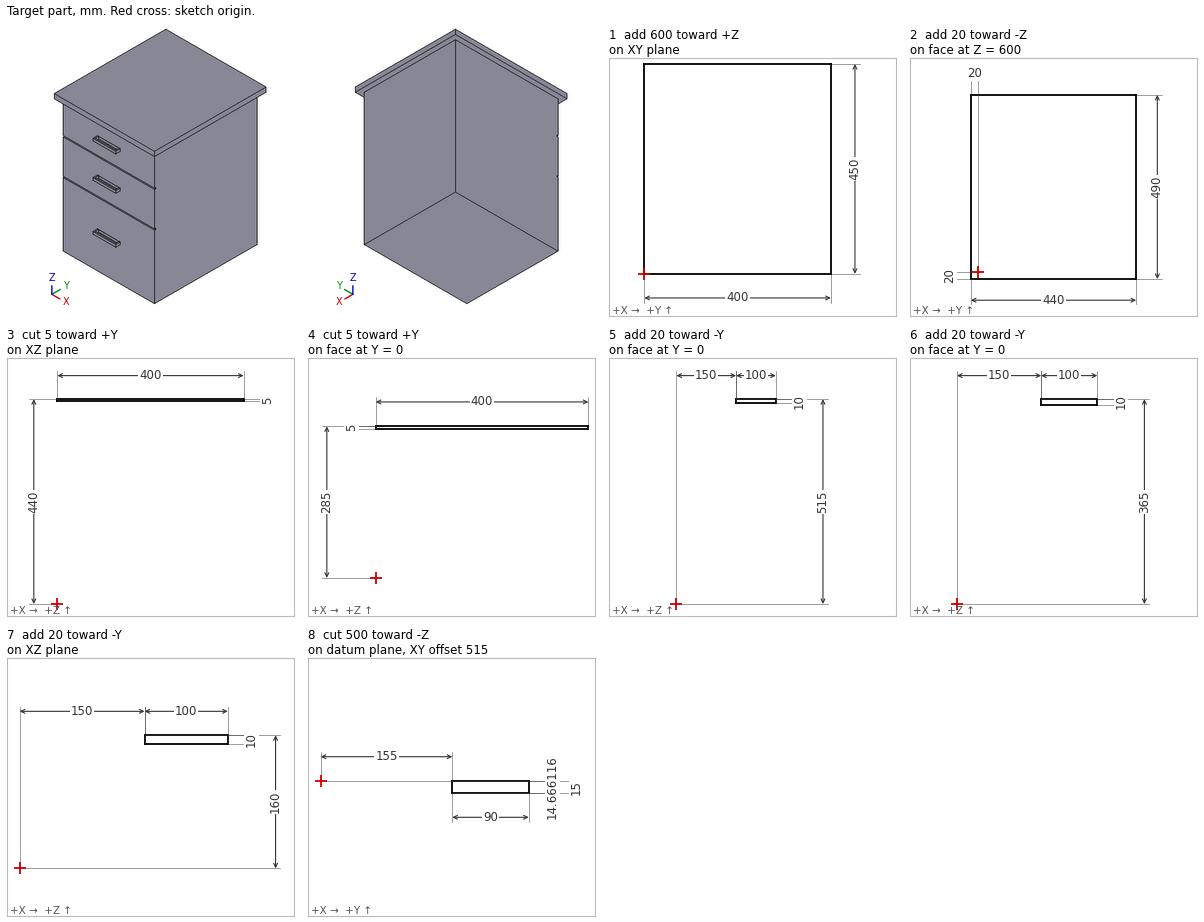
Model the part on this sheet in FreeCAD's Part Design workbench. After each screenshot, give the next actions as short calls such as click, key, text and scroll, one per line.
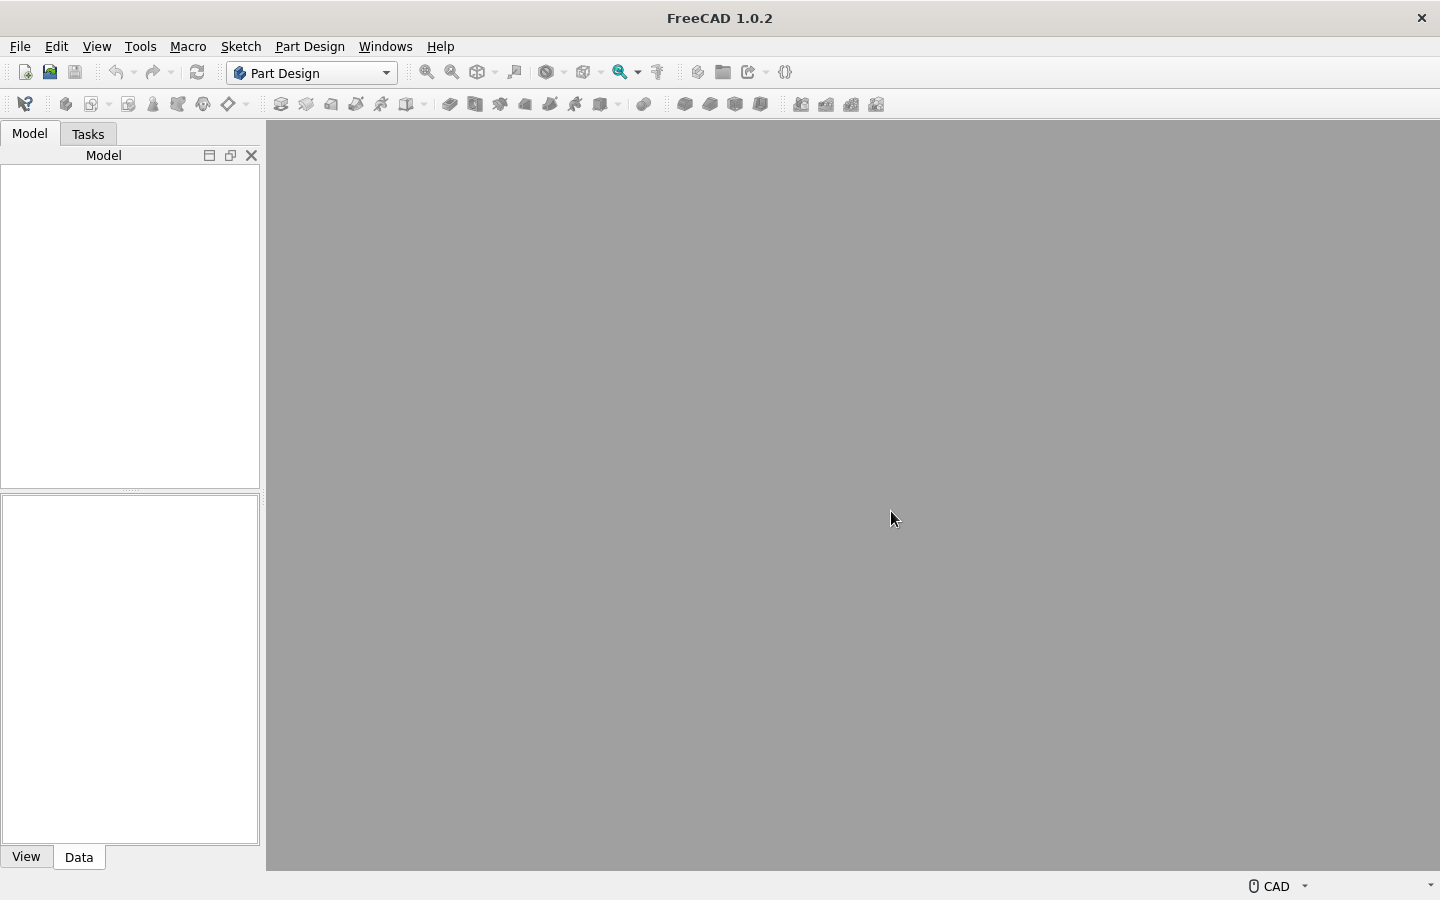
click(25, 72)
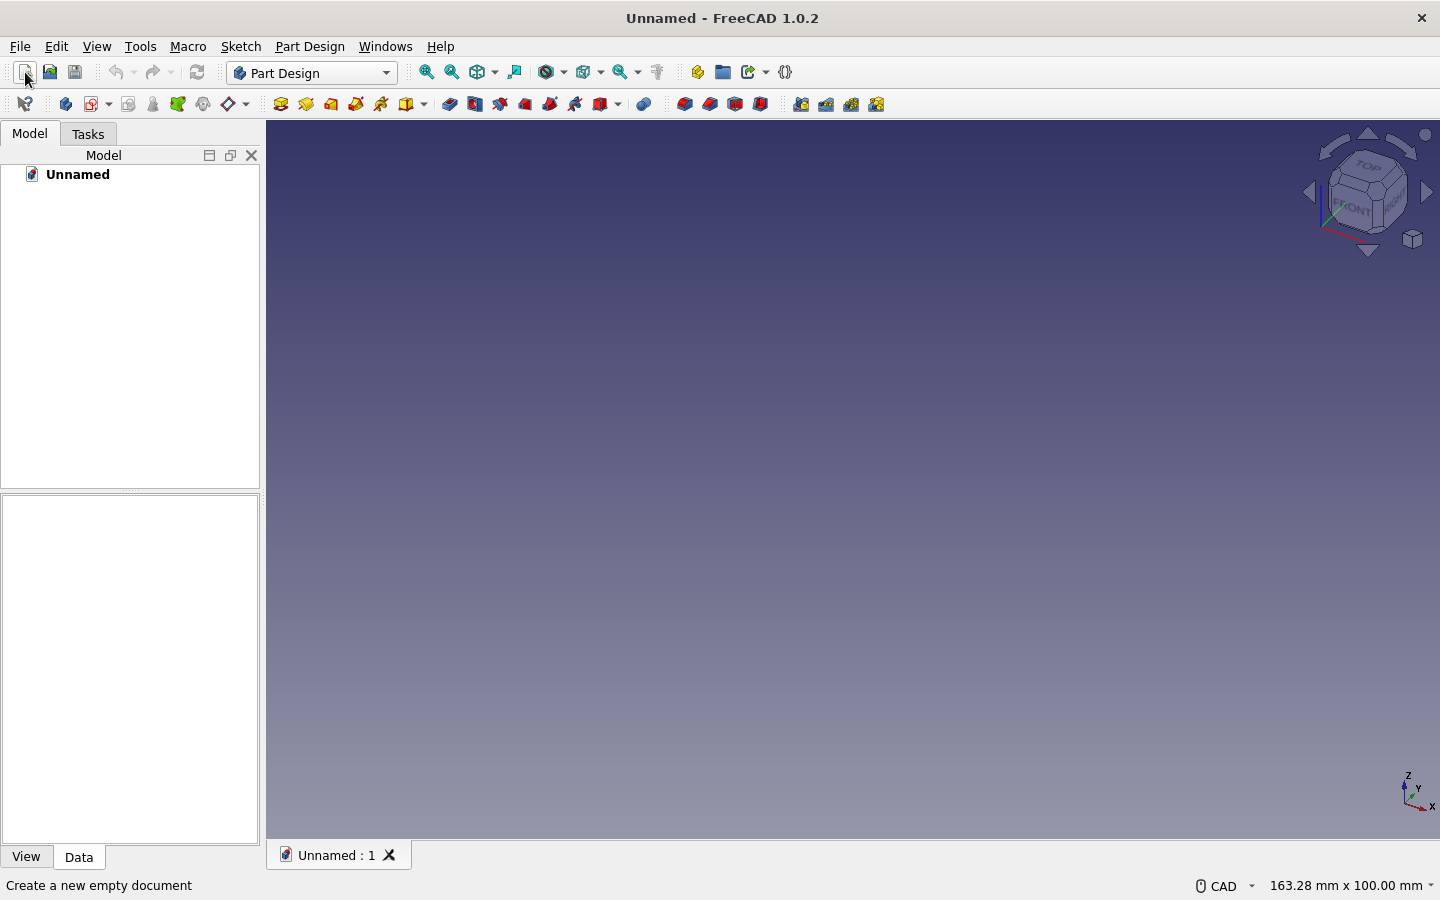
click(90, 104)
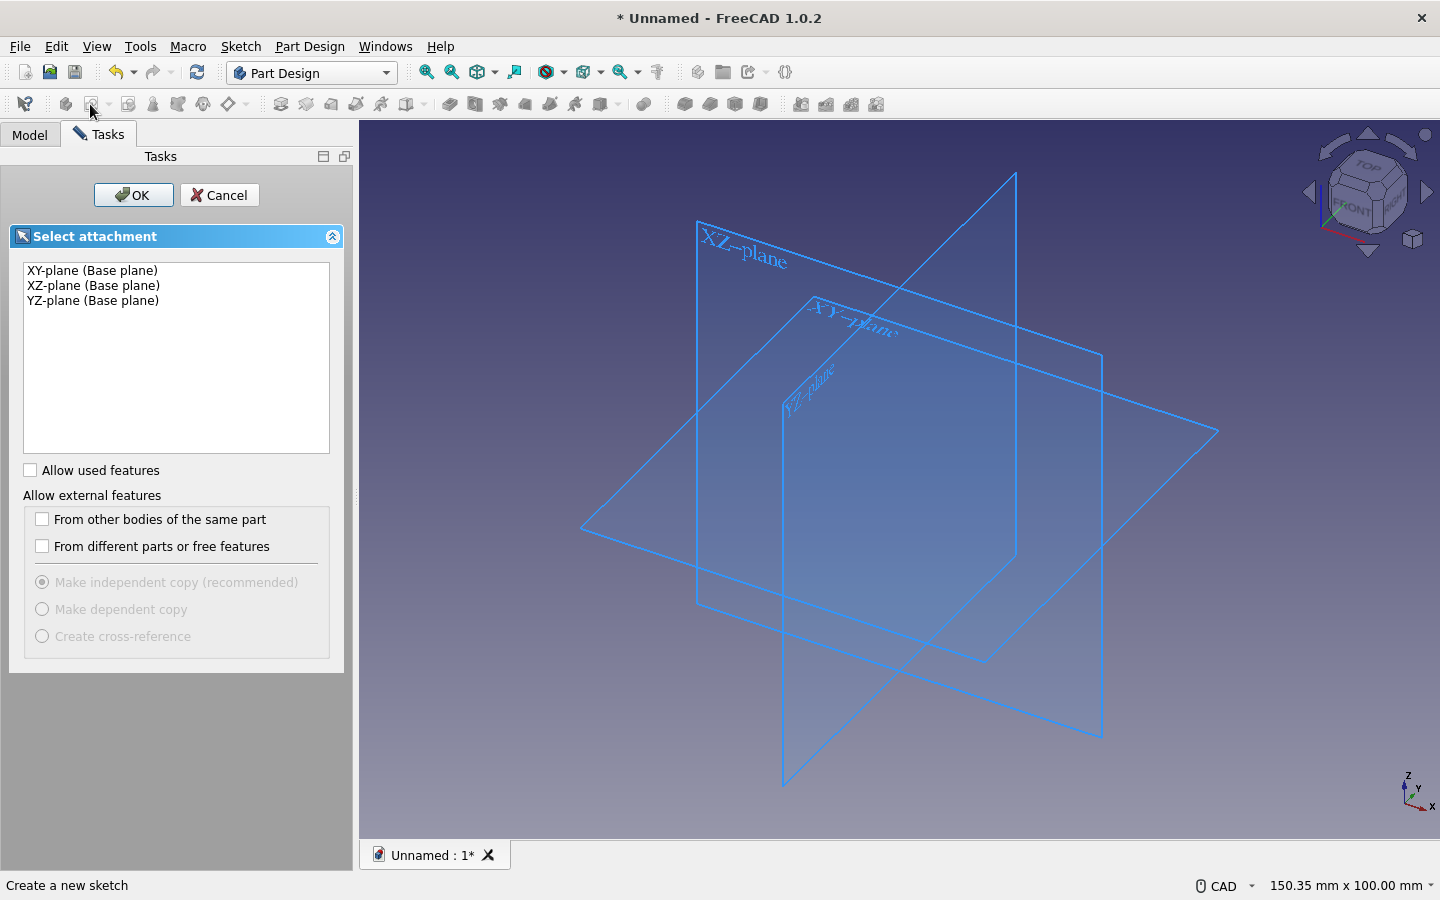
click(84, 270)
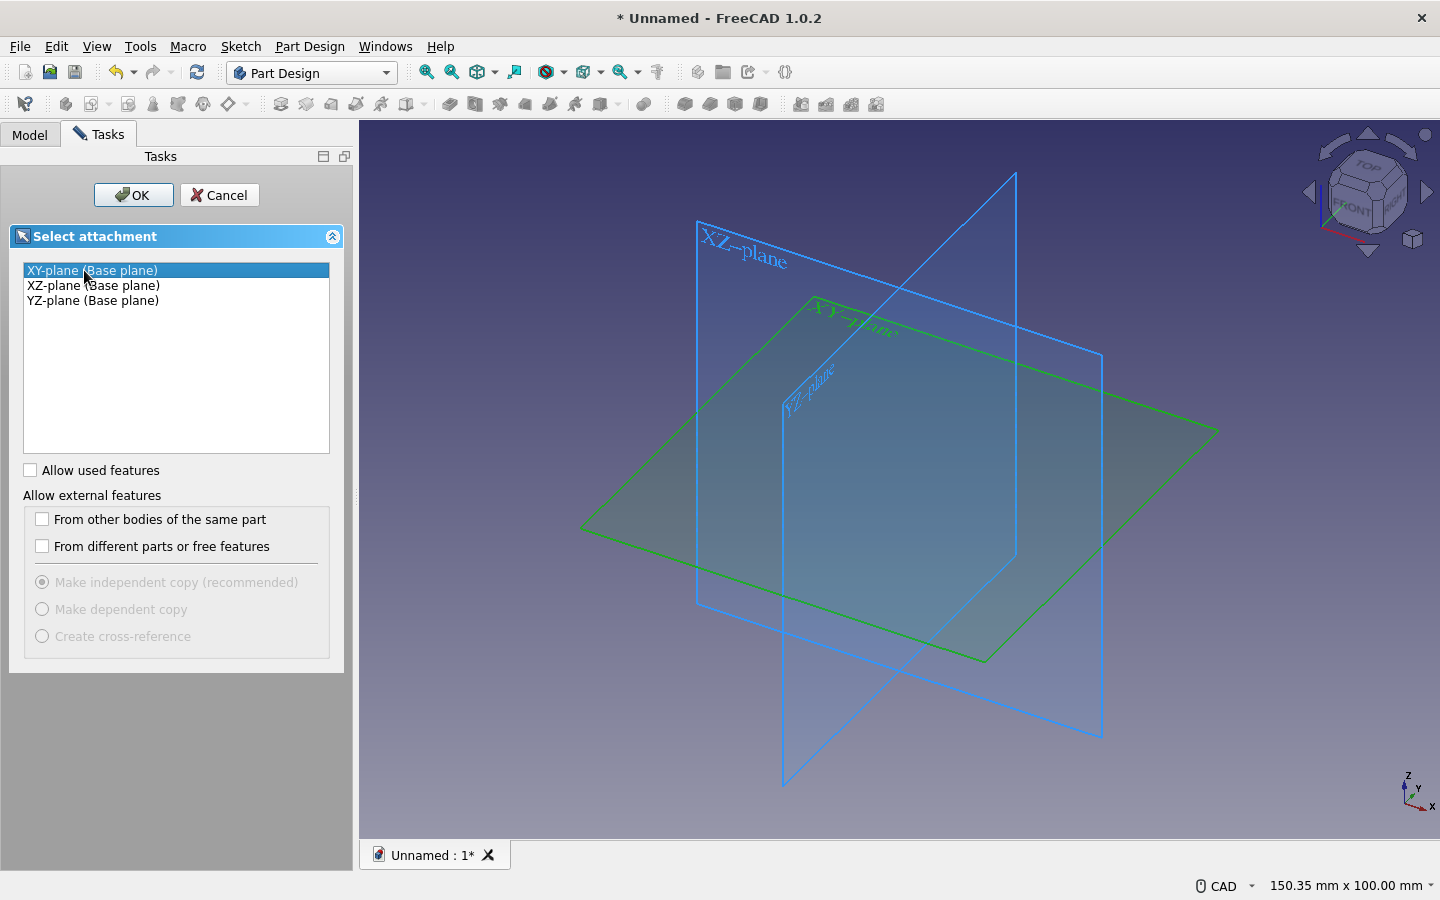
click(134, 195)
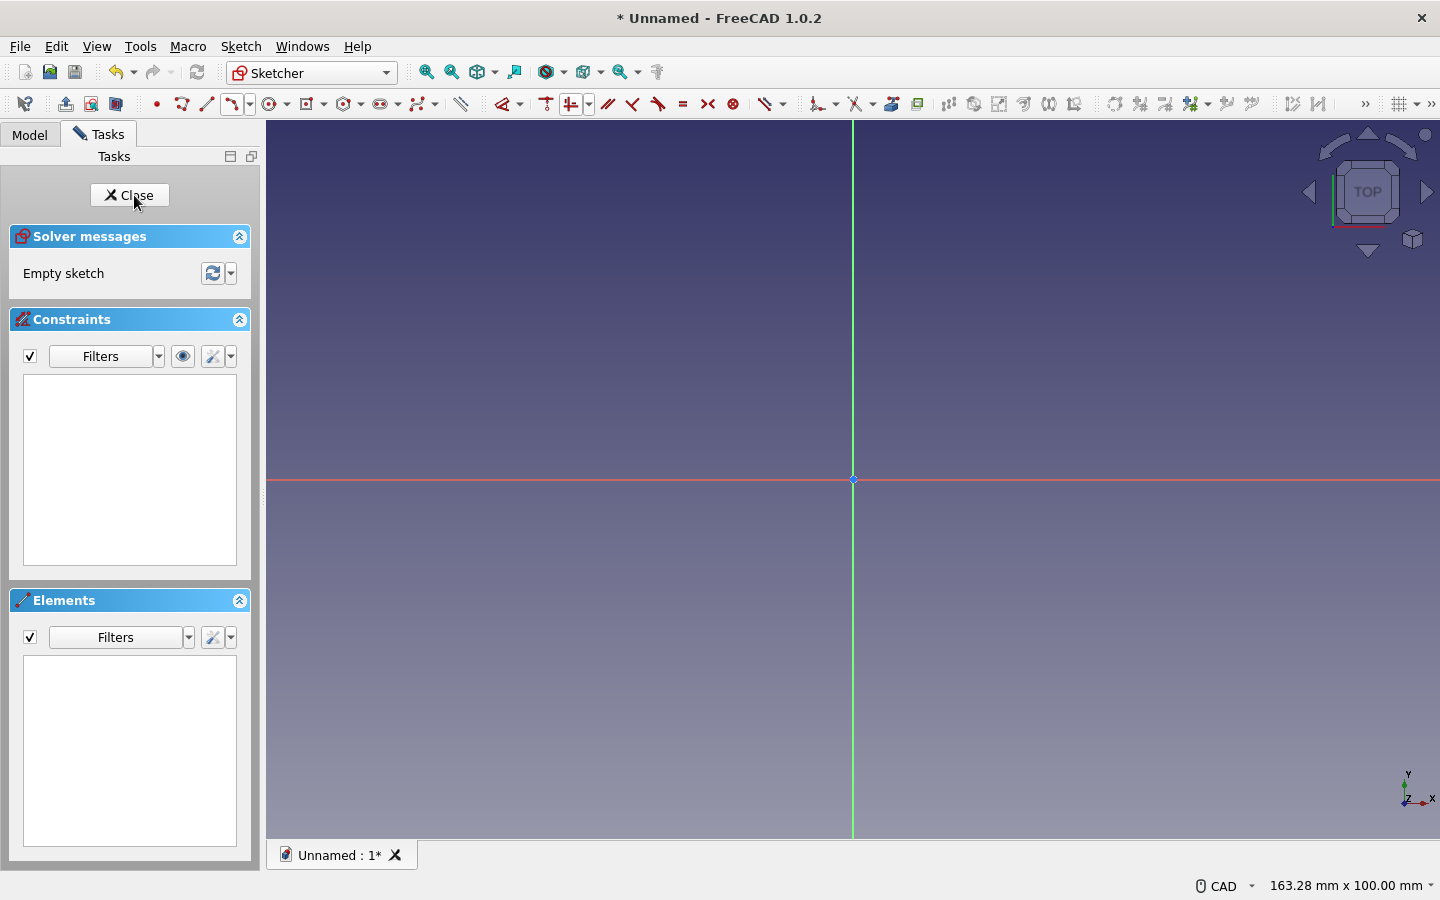
scroll(549, 733, down, 10)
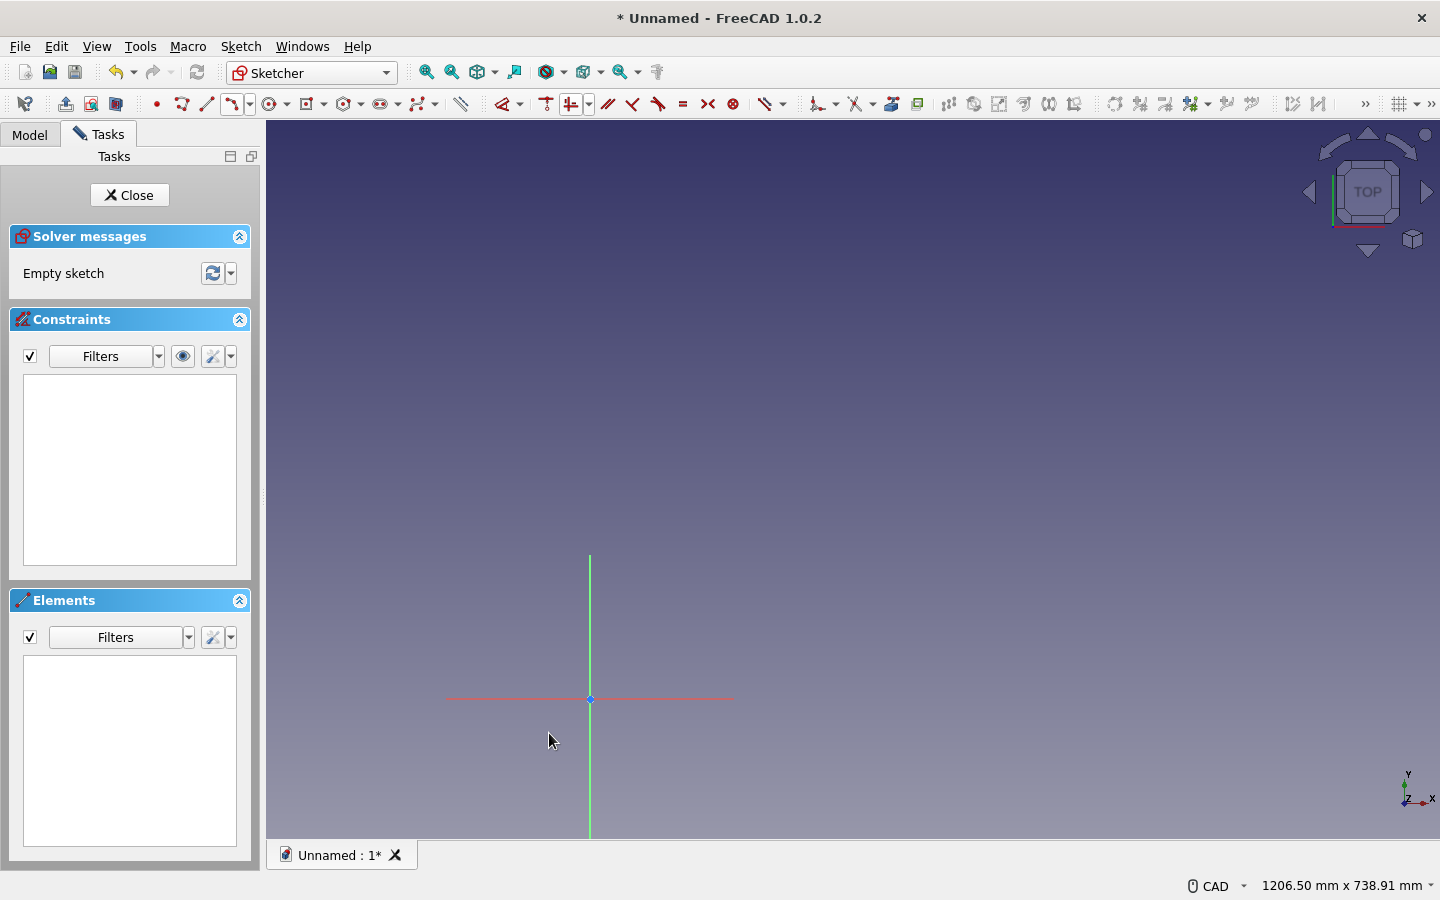
click(324, 104)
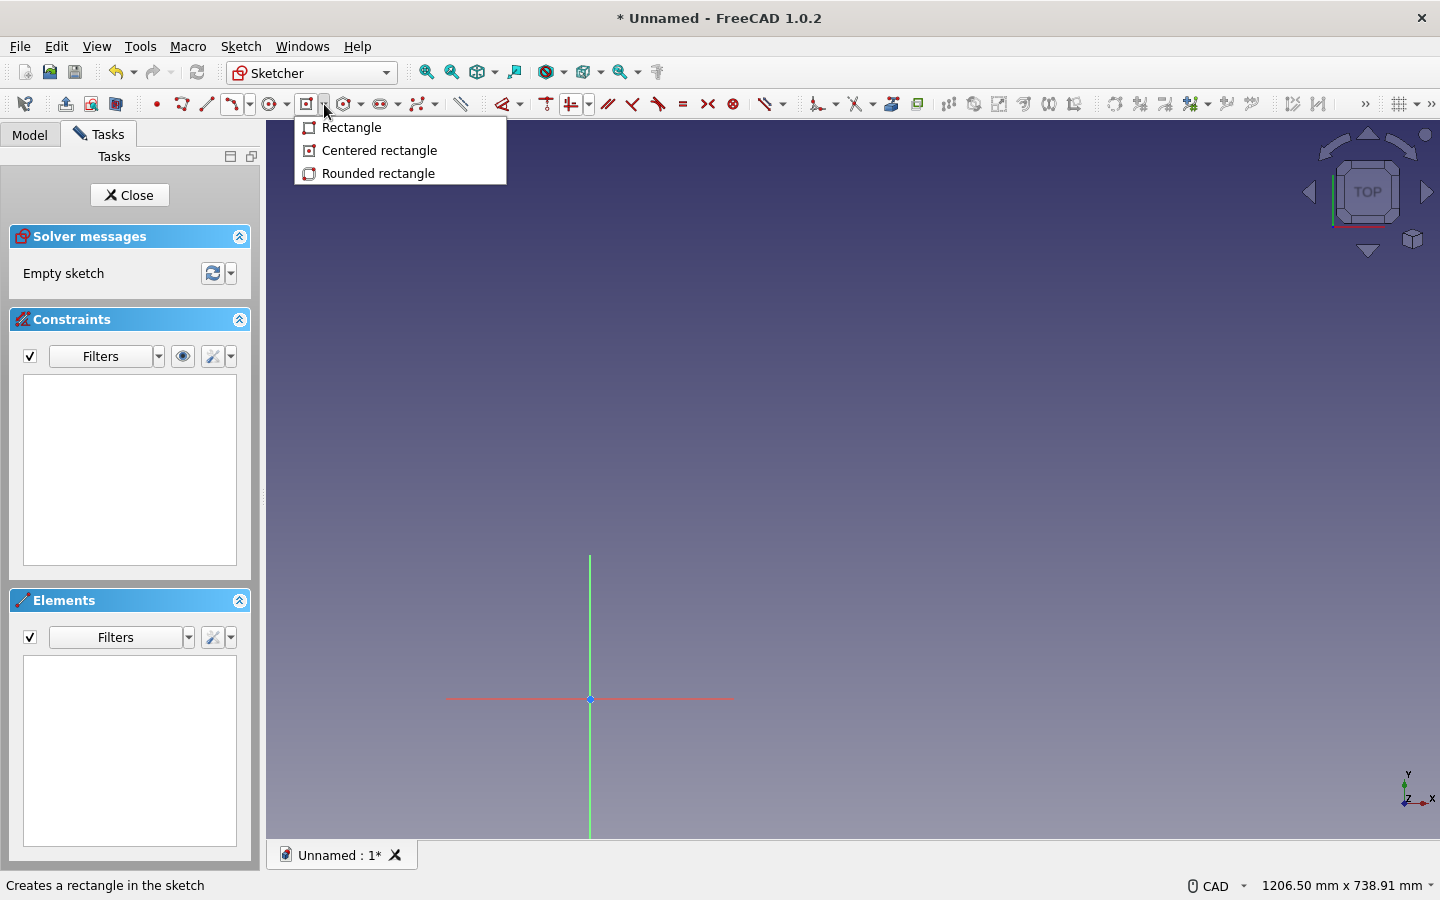
click(400, 128)